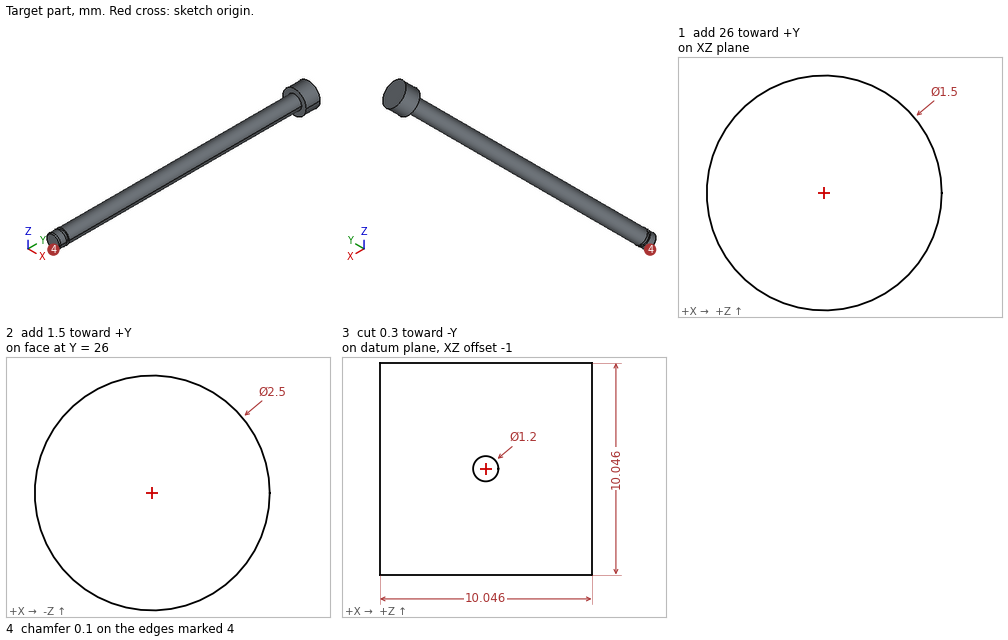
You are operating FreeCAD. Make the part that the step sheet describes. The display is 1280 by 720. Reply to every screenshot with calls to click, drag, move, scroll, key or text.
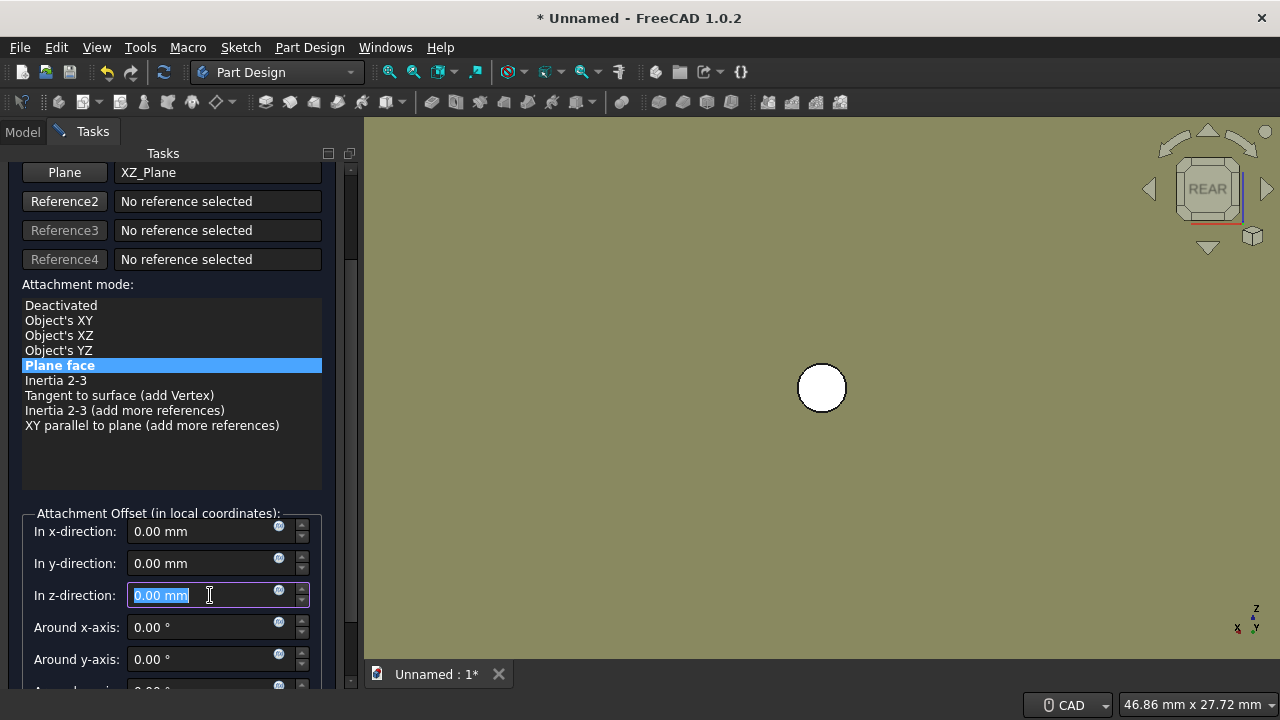
text(-1)
key(Tab)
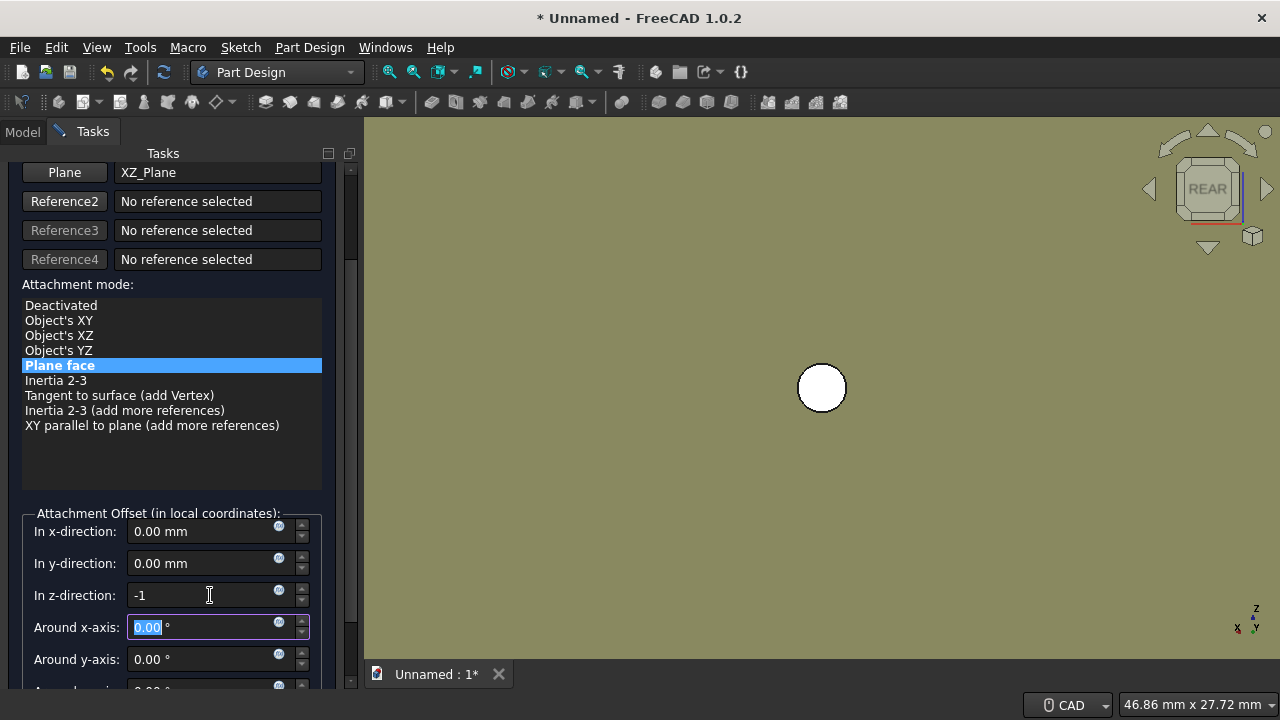
scroll(351, 426, up, 3)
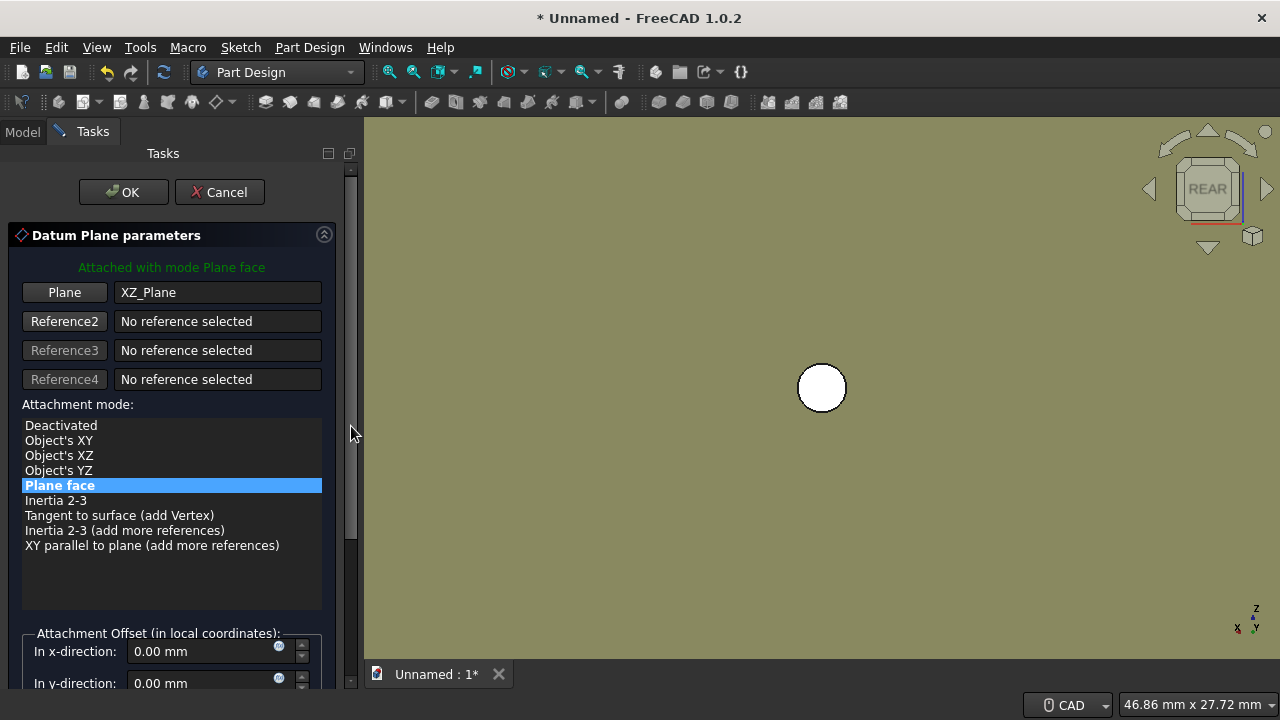
click(124, 192)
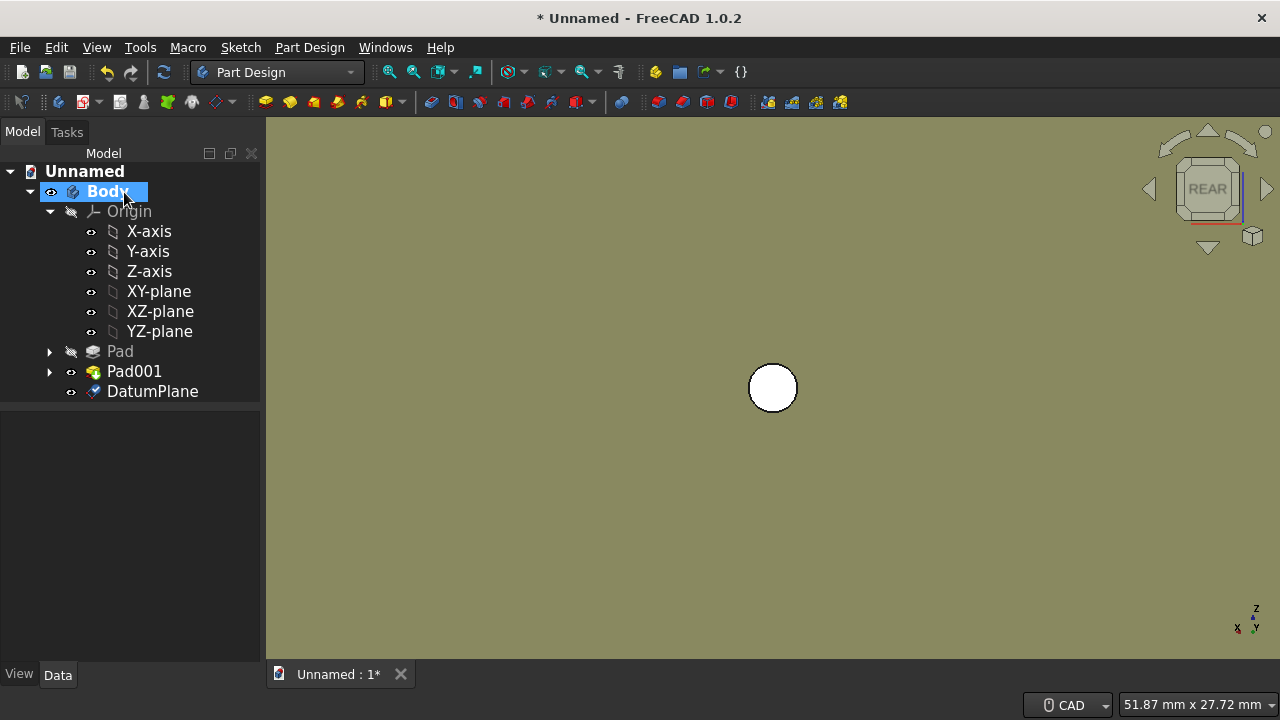
click(116, 392)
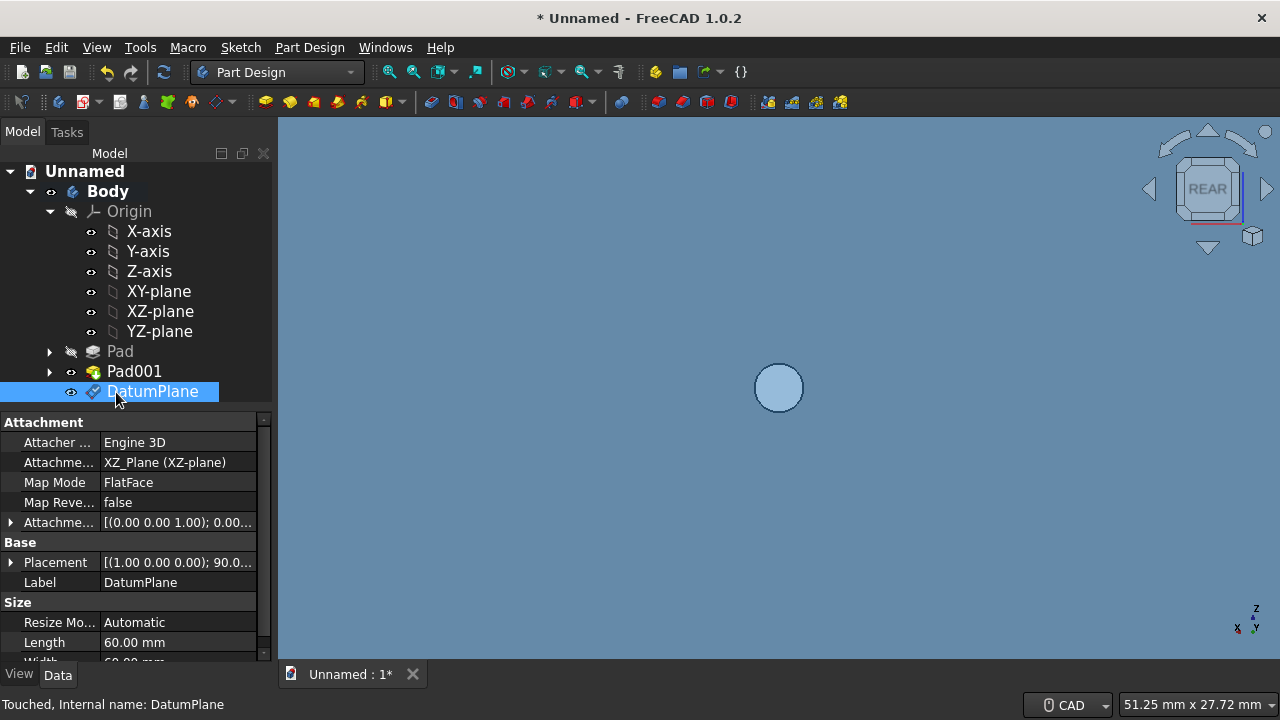
click(84, 102)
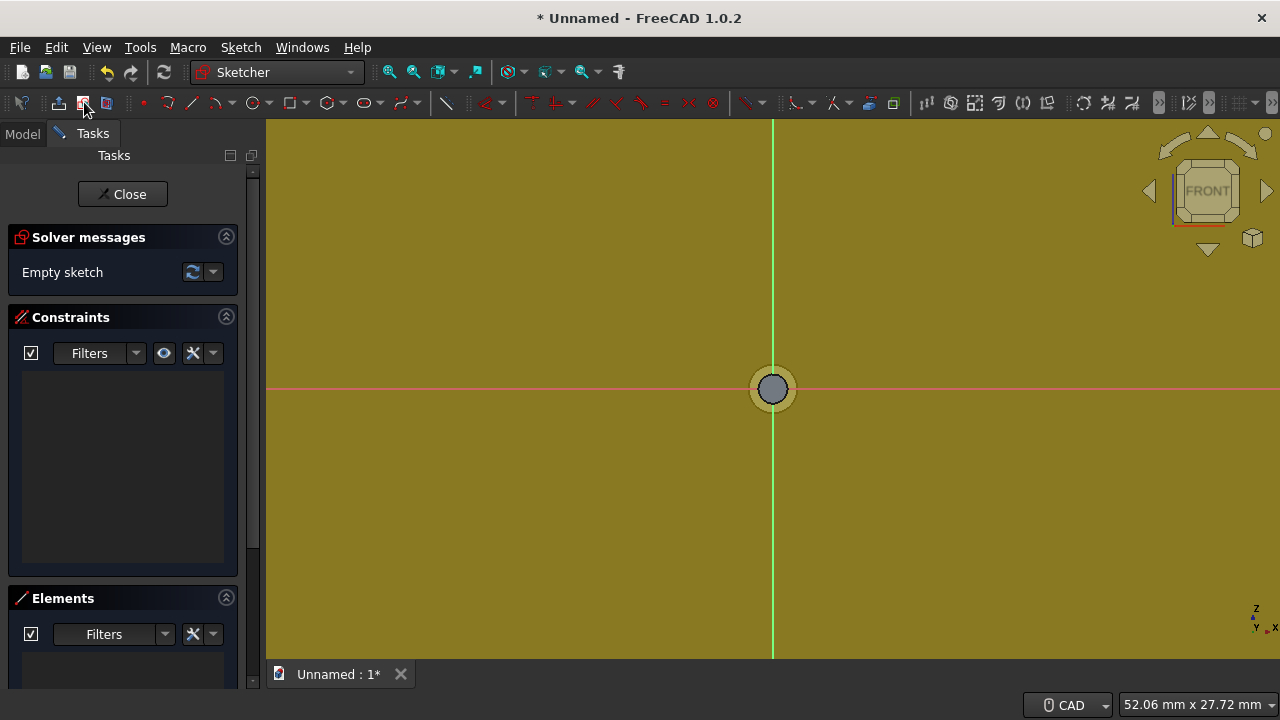
click(108, 104)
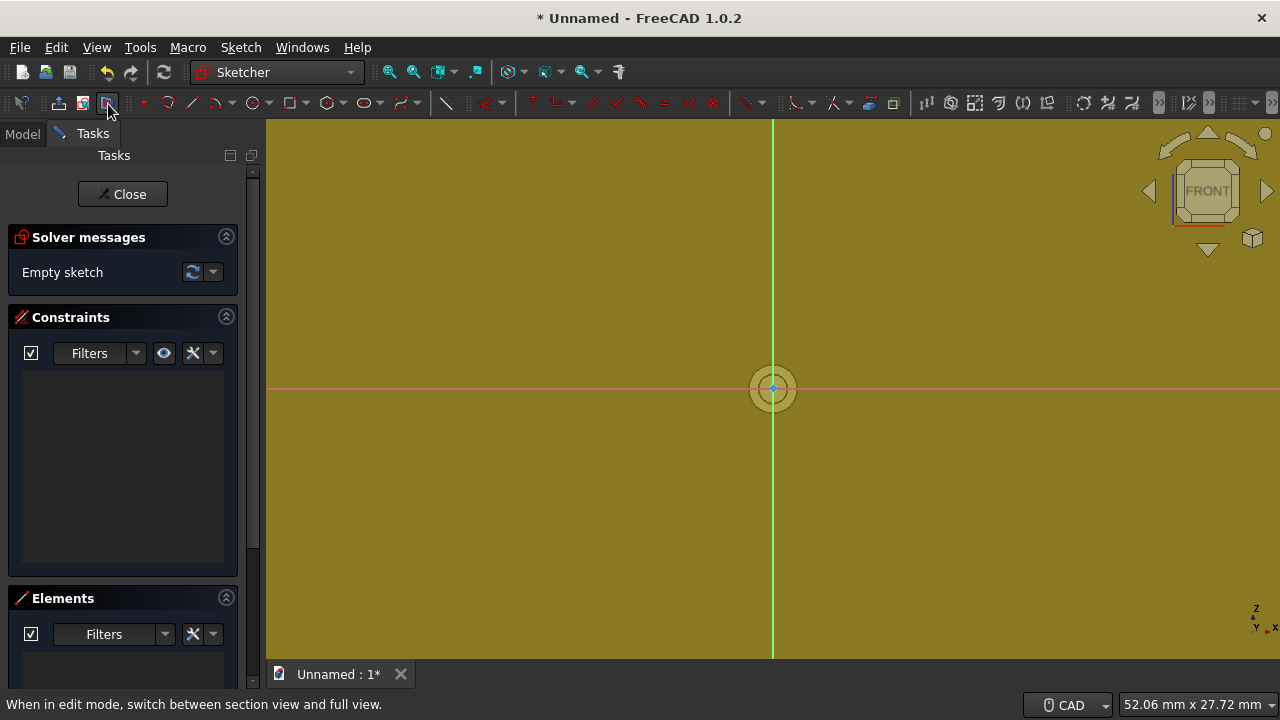
scroll(856, 389, up, 3)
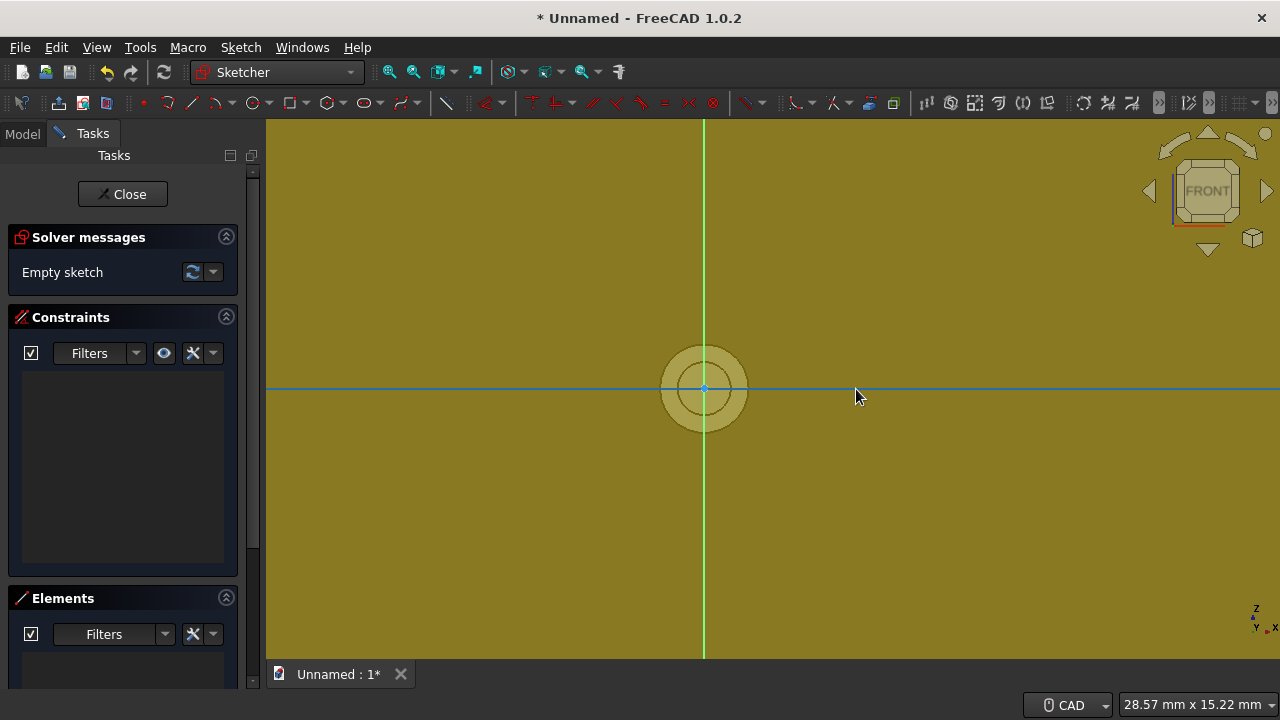
click(308, 104)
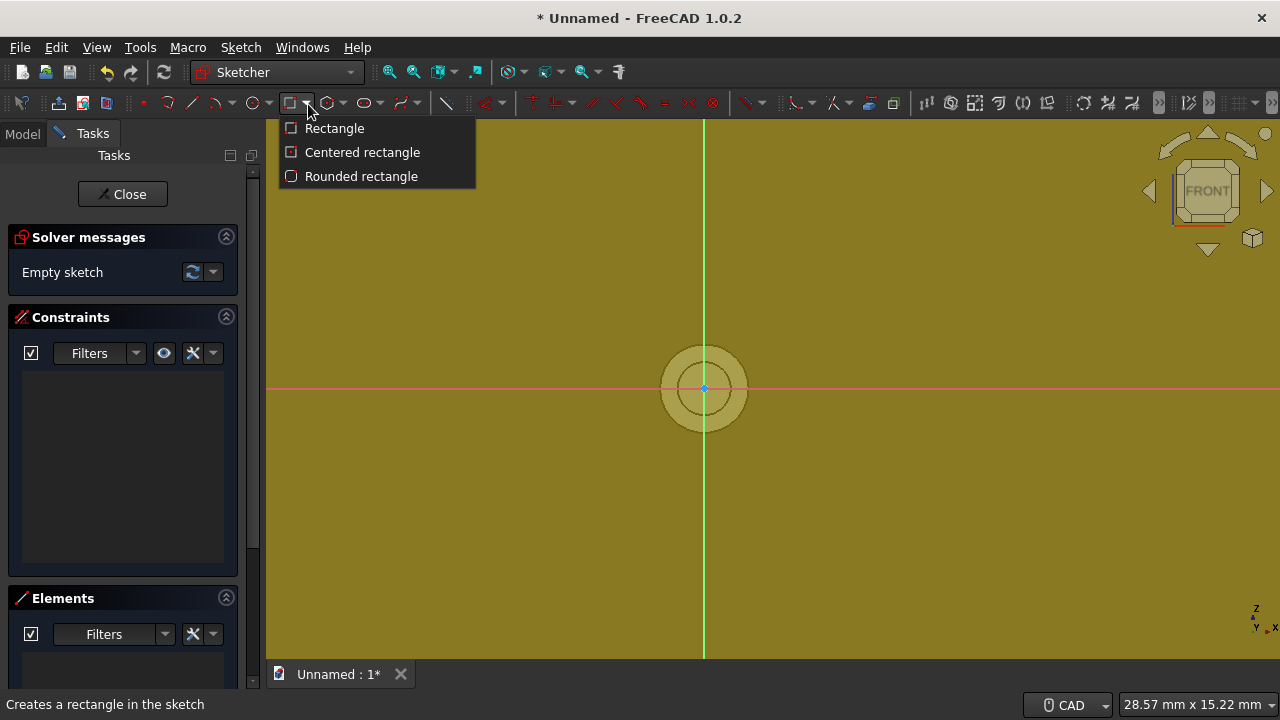
click(378, 152)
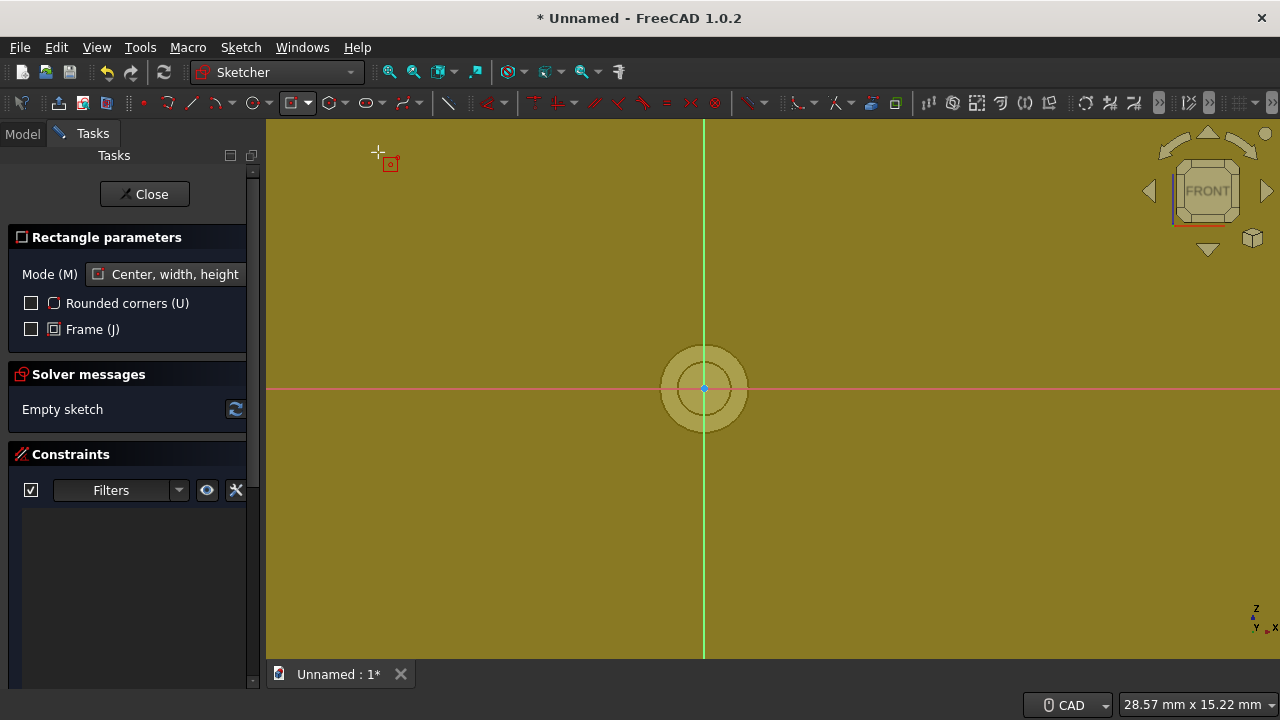
click(704, 389)
move(883, 210)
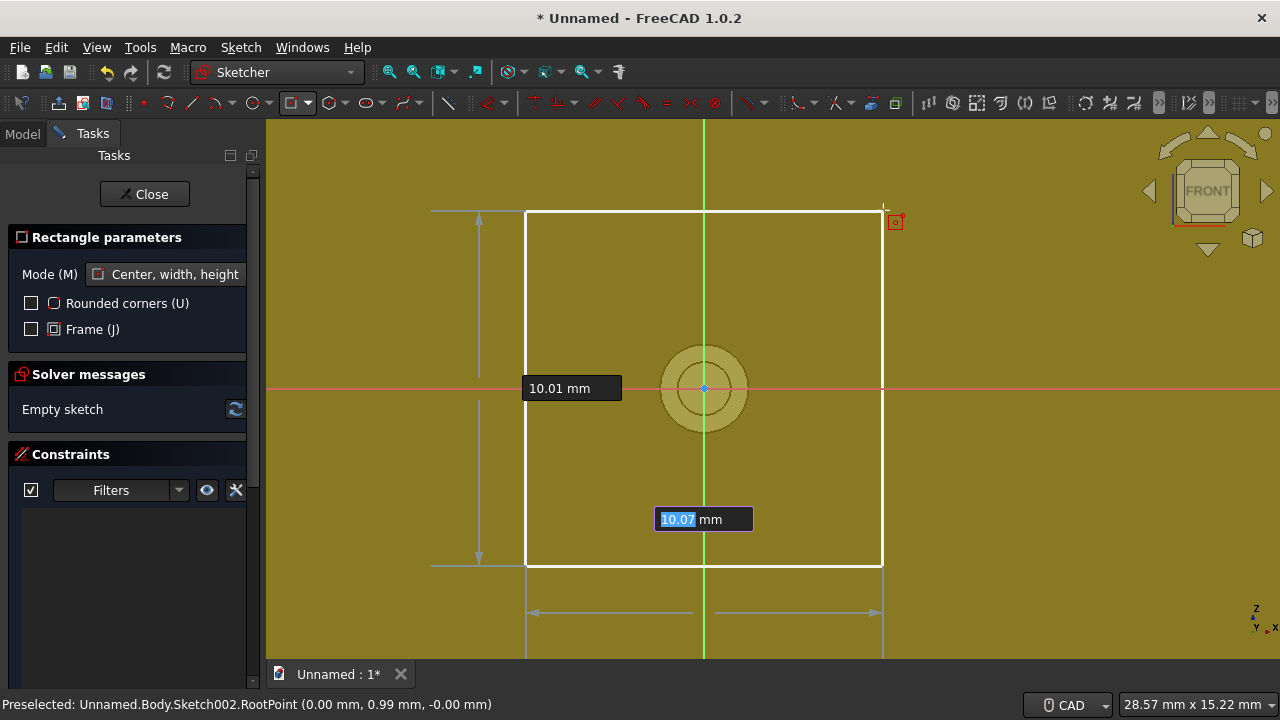
text(10.046)
key(Tab)
text(10.046)
key(Return)